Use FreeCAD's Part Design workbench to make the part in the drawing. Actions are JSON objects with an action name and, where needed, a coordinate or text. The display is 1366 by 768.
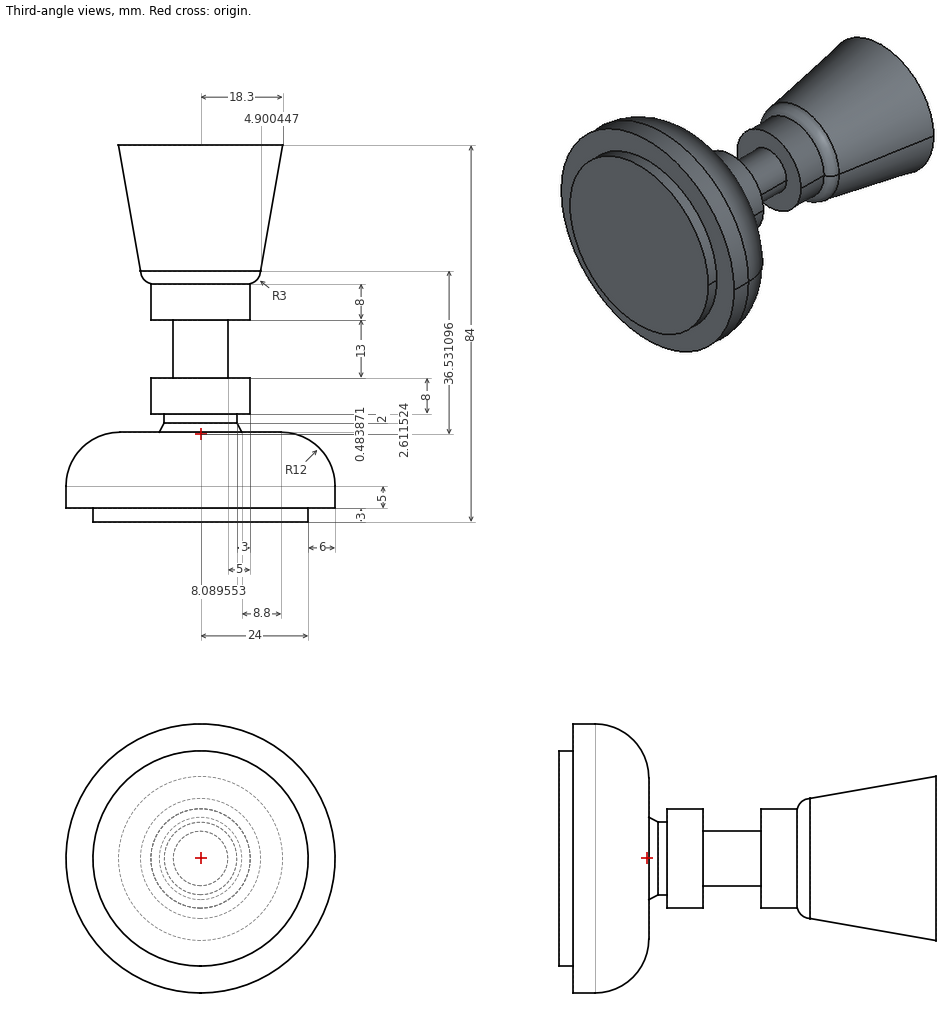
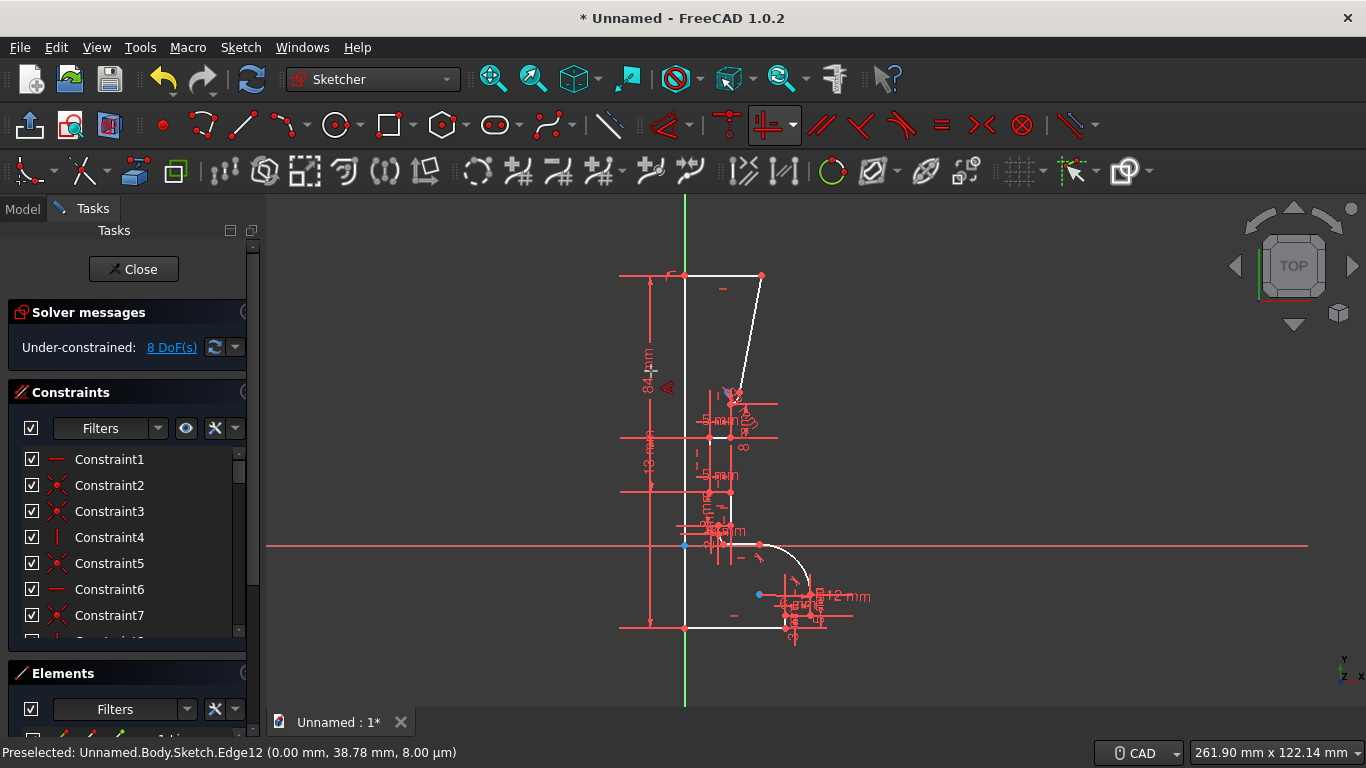
{"action": "left_click", "coordinate": [715, 628]}
{"action": "left_click", "coordinate": [735, 662]}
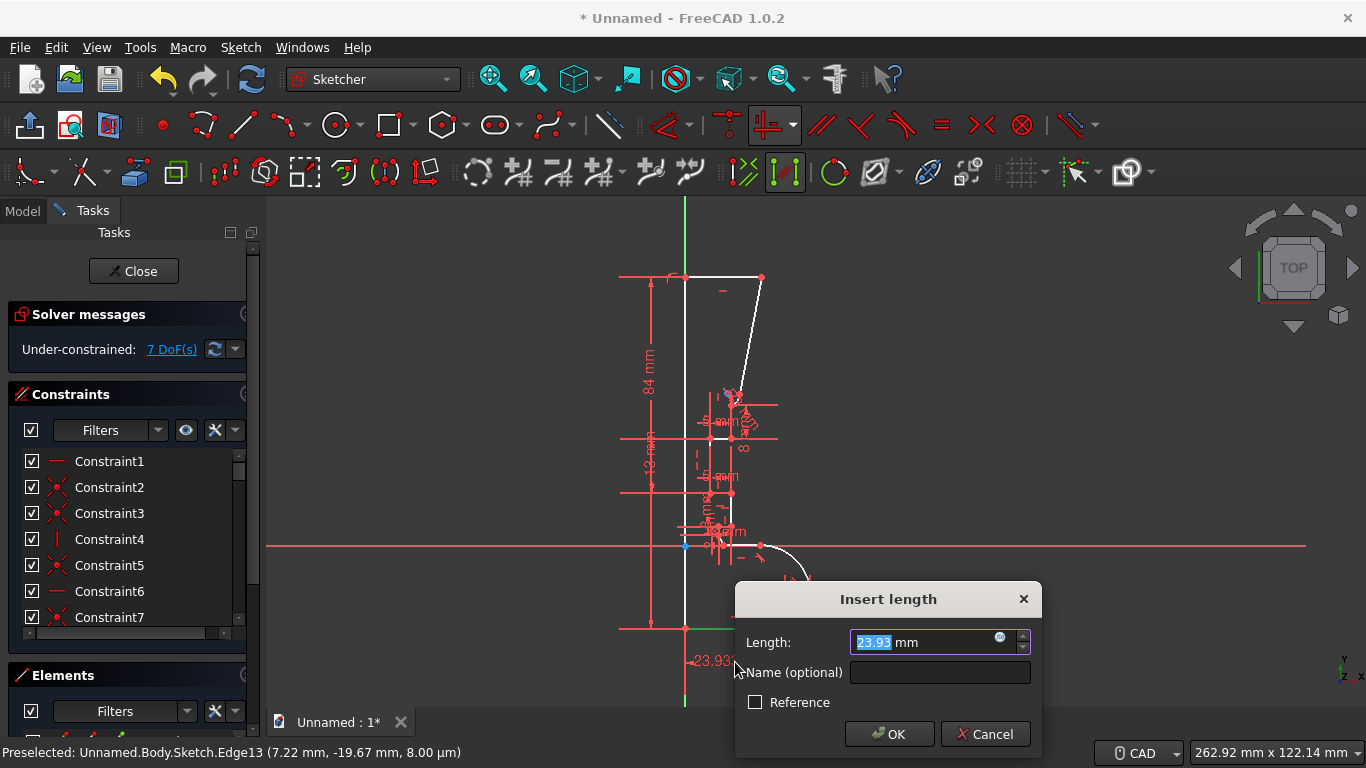
{"action": "type", "text": "24"}
{"action": "key", "text": "Return"}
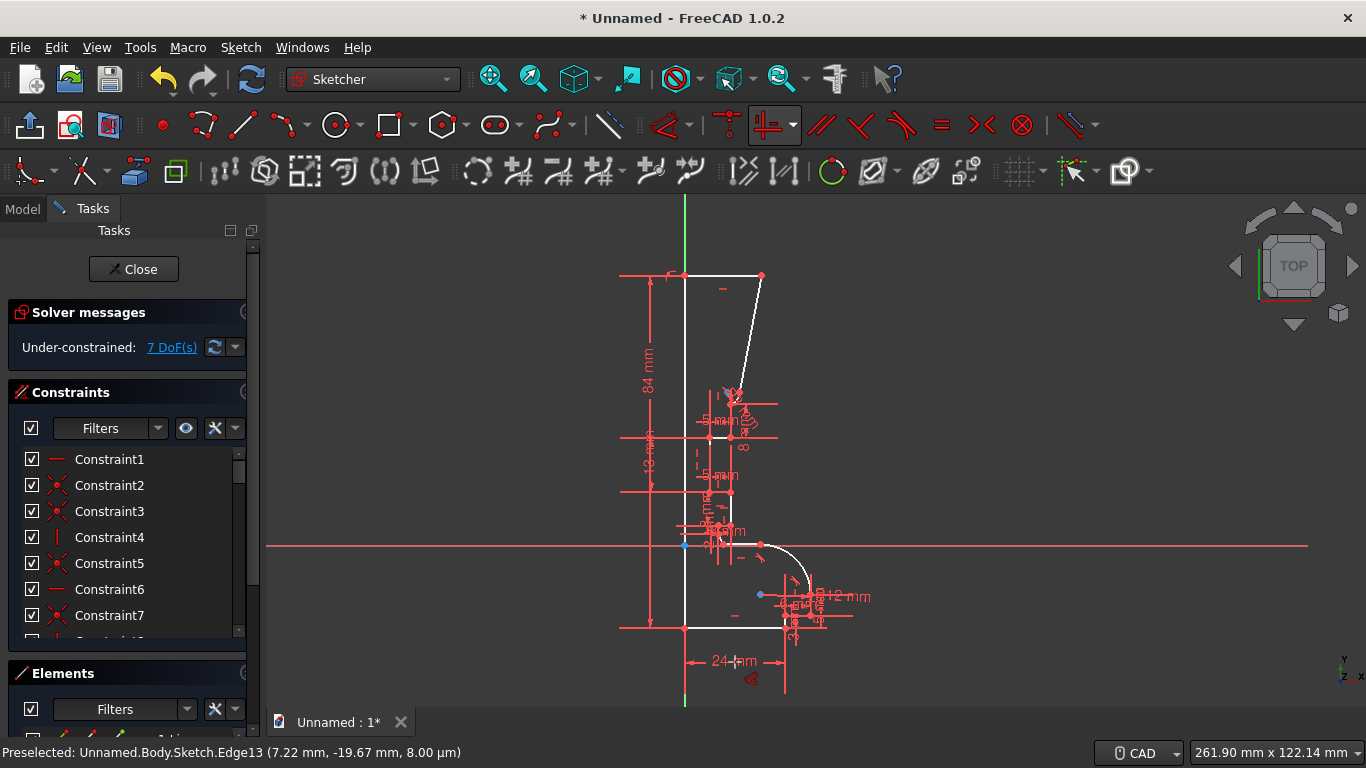
{"action": "scroll", "coordinate": [749, 544], "scroll_direction": "up", "scroll_amount": 2}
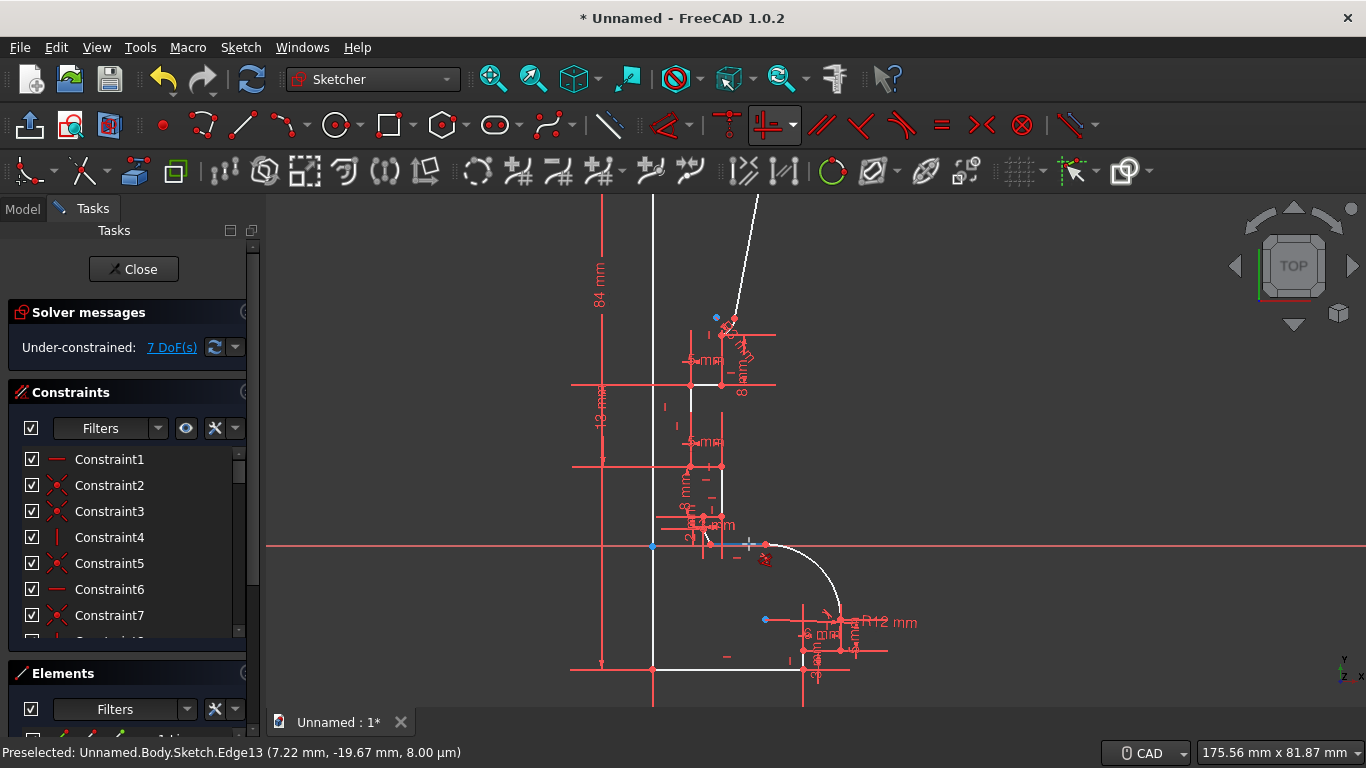
{"action": "left_click", "coordinate": [749, 544]}
{"action": "left_click", "coordinate": [738, 578]}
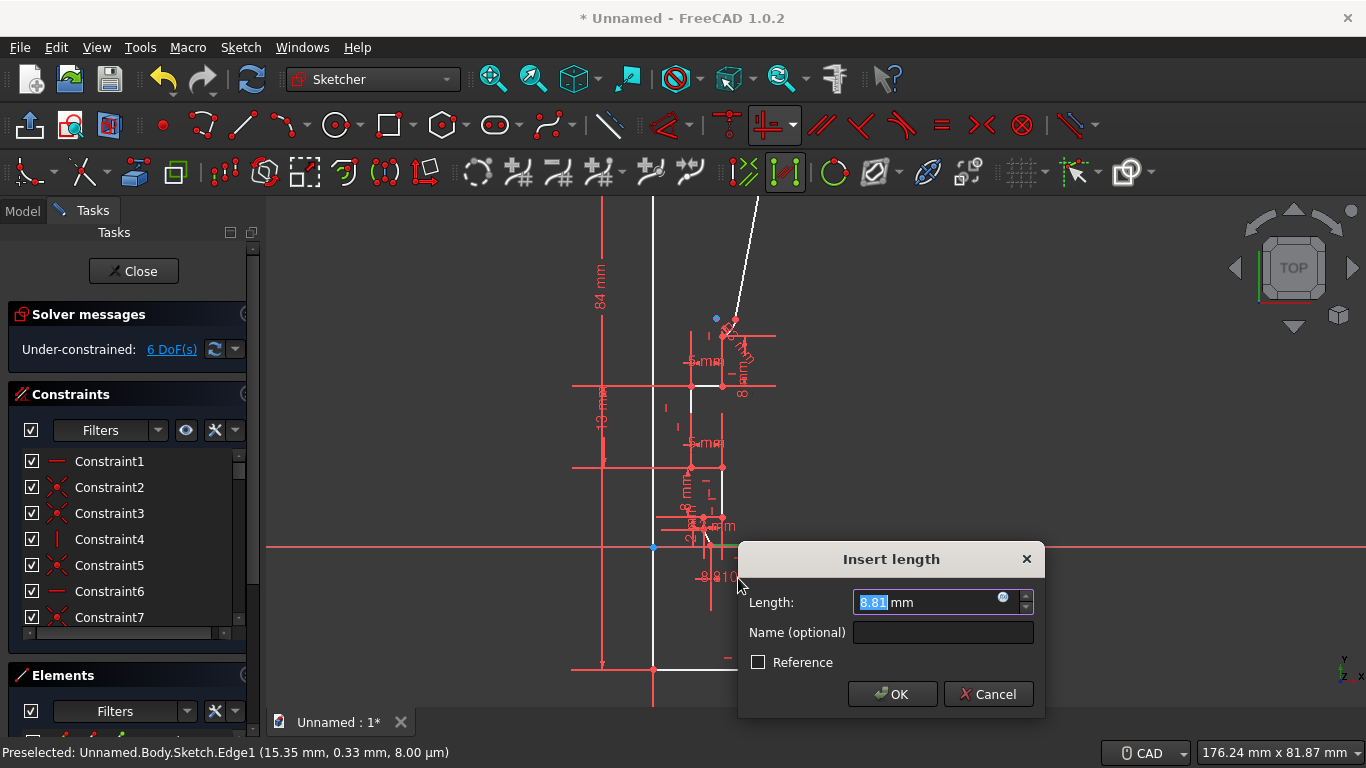
{"action": "type", "text": "8.8"}
{"action": "key", "text": "Return"}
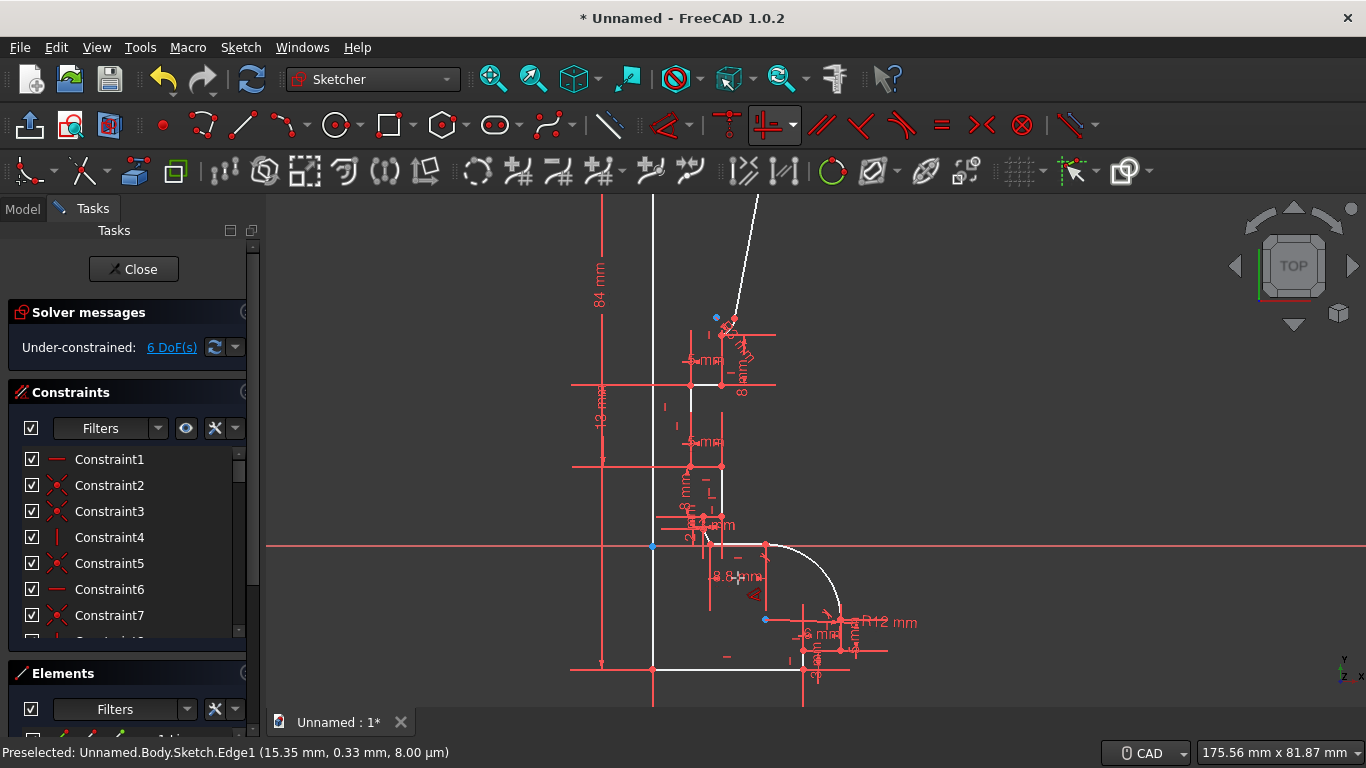
{"action": "scroll", "coordinate": [749, 542], "scroll_direction": "down", "scroll_amount": 2}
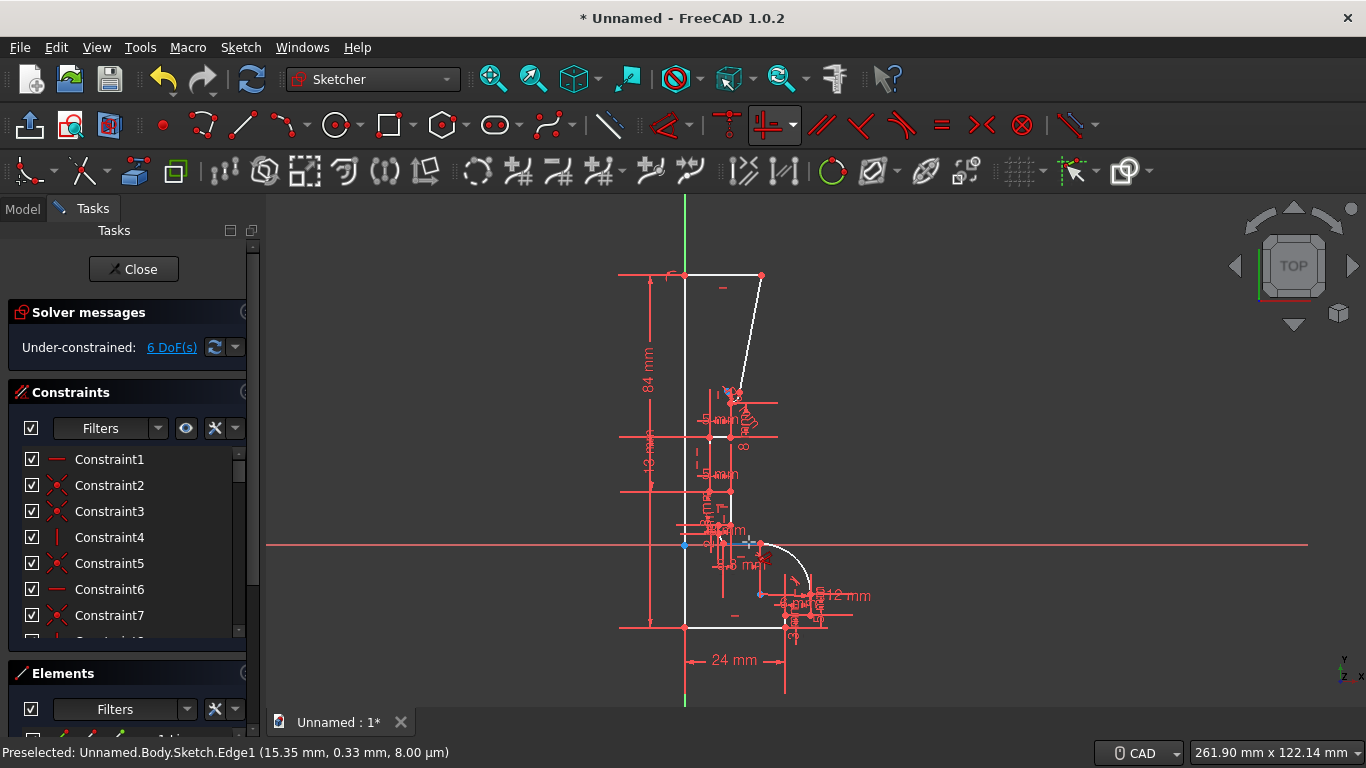
{"action": "left_click", "coordinate": [739, 275]}
{"action": "left_click", "coordinate": [723, 241]}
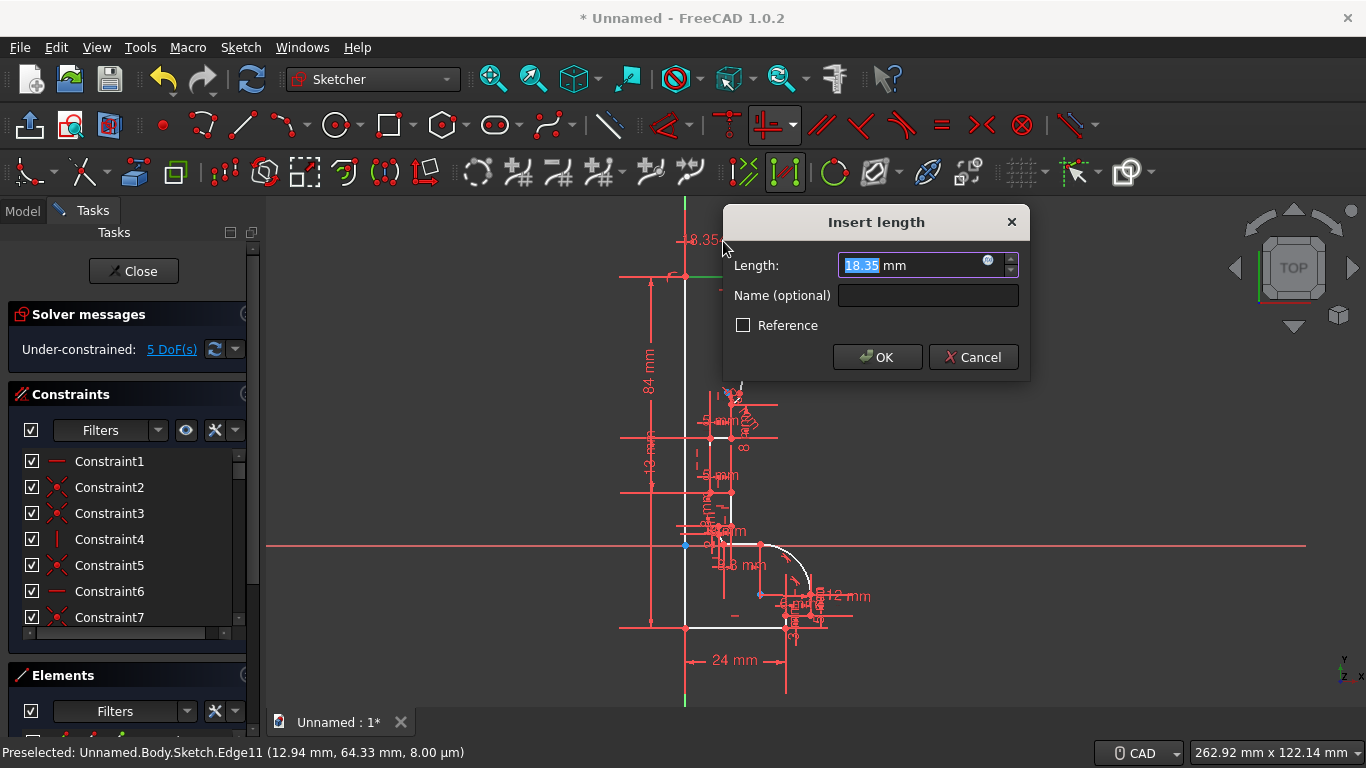
{"action": "type", "text": "18.3"}
{"action": "key", "text": "Return"}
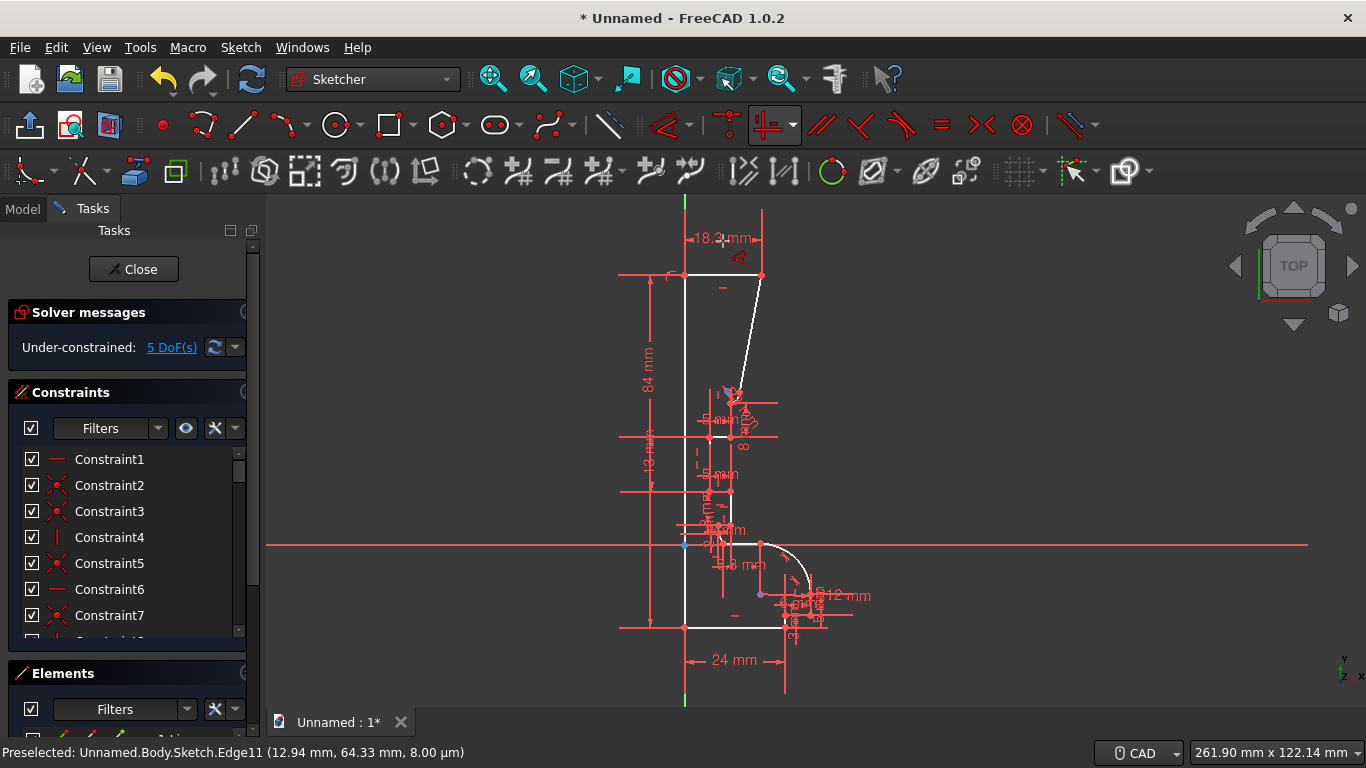
{"action": "scroll", "coordinate": [760, 544], "scroll_direction": "up", "scroll_amount": 15}